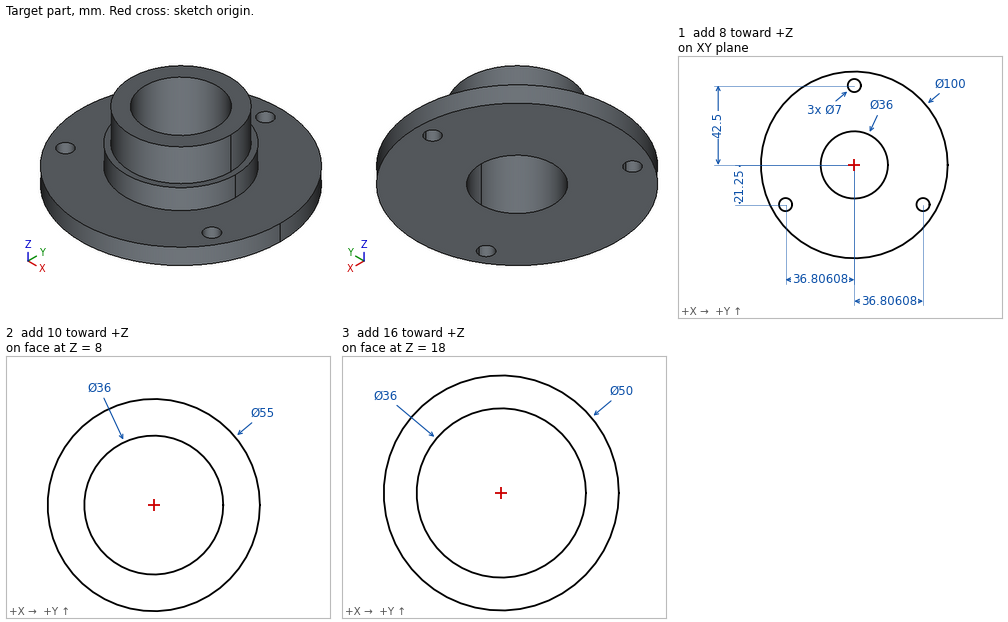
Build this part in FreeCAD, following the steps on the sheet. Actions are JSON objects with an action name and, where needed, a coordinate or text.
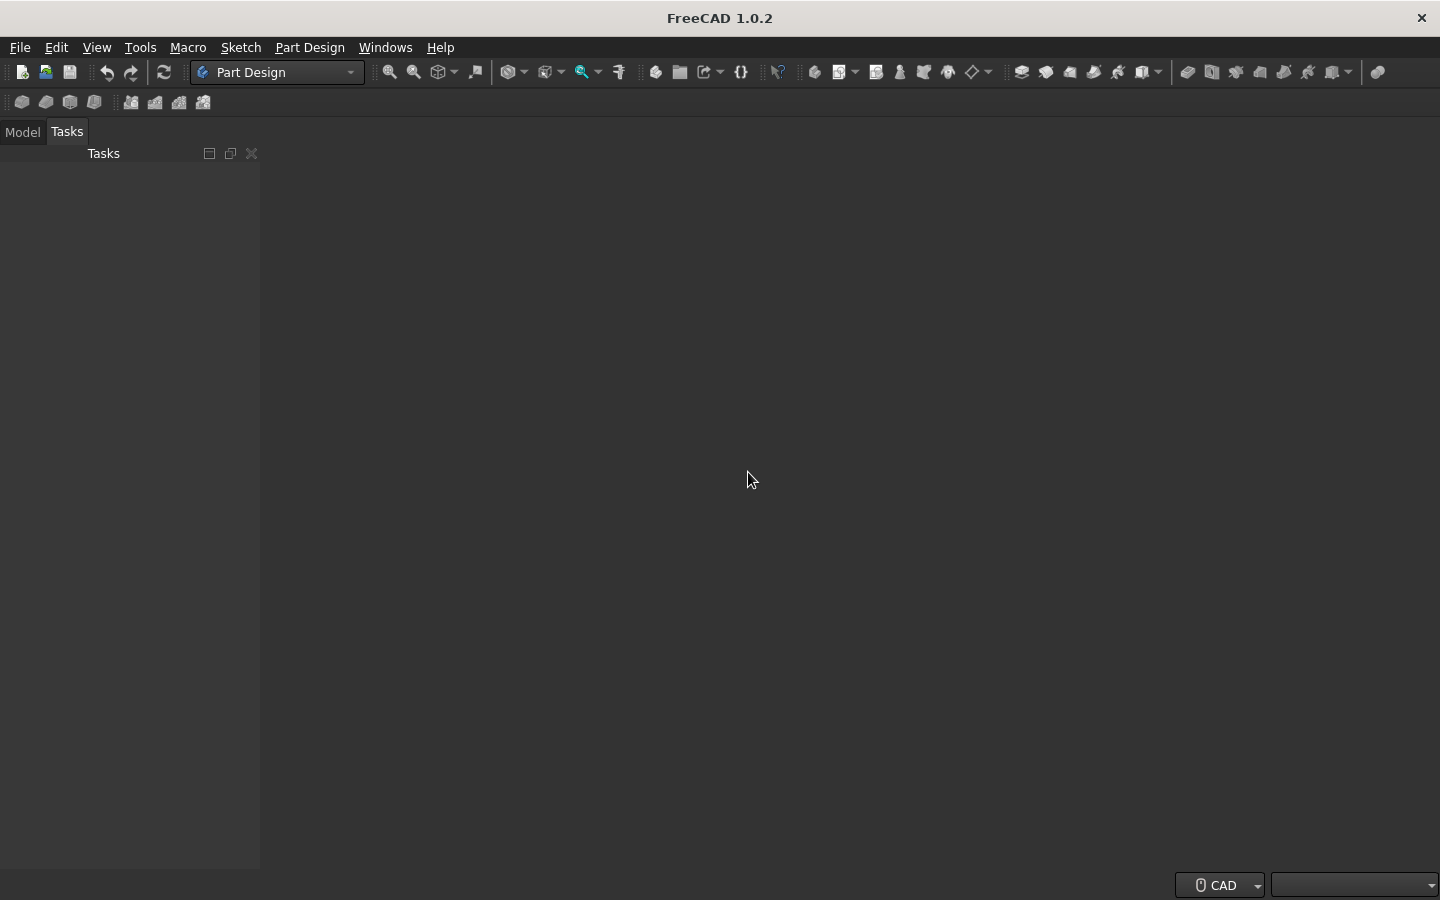
{"action": "left_click", "coordinate": [22, 72]}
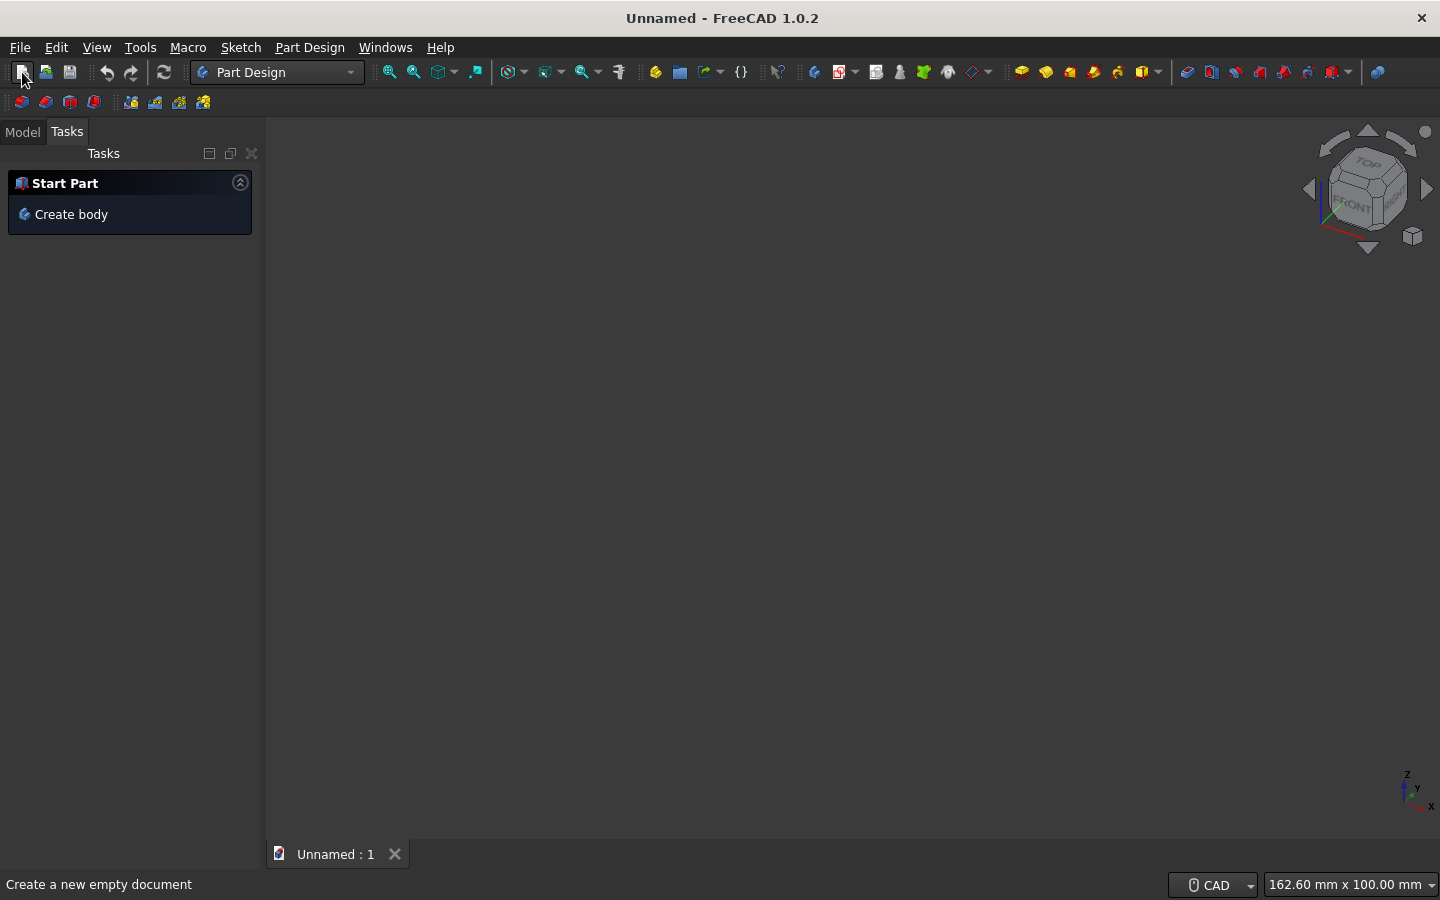
{"action": "left_click", "coordinate": [840, 72]}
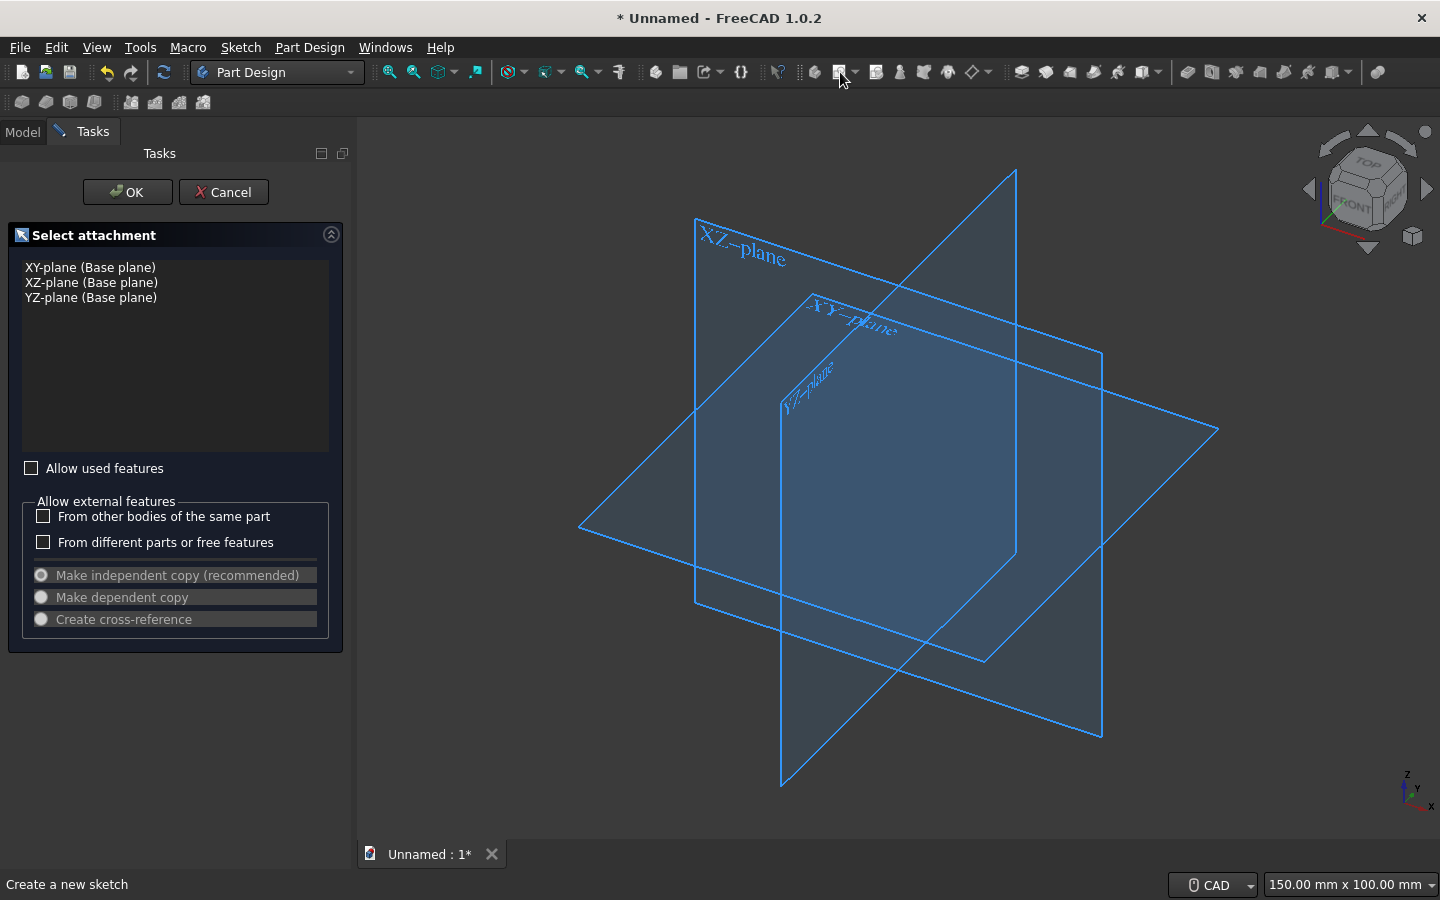
{"action": "left_click", "coordinate": [82, 268]}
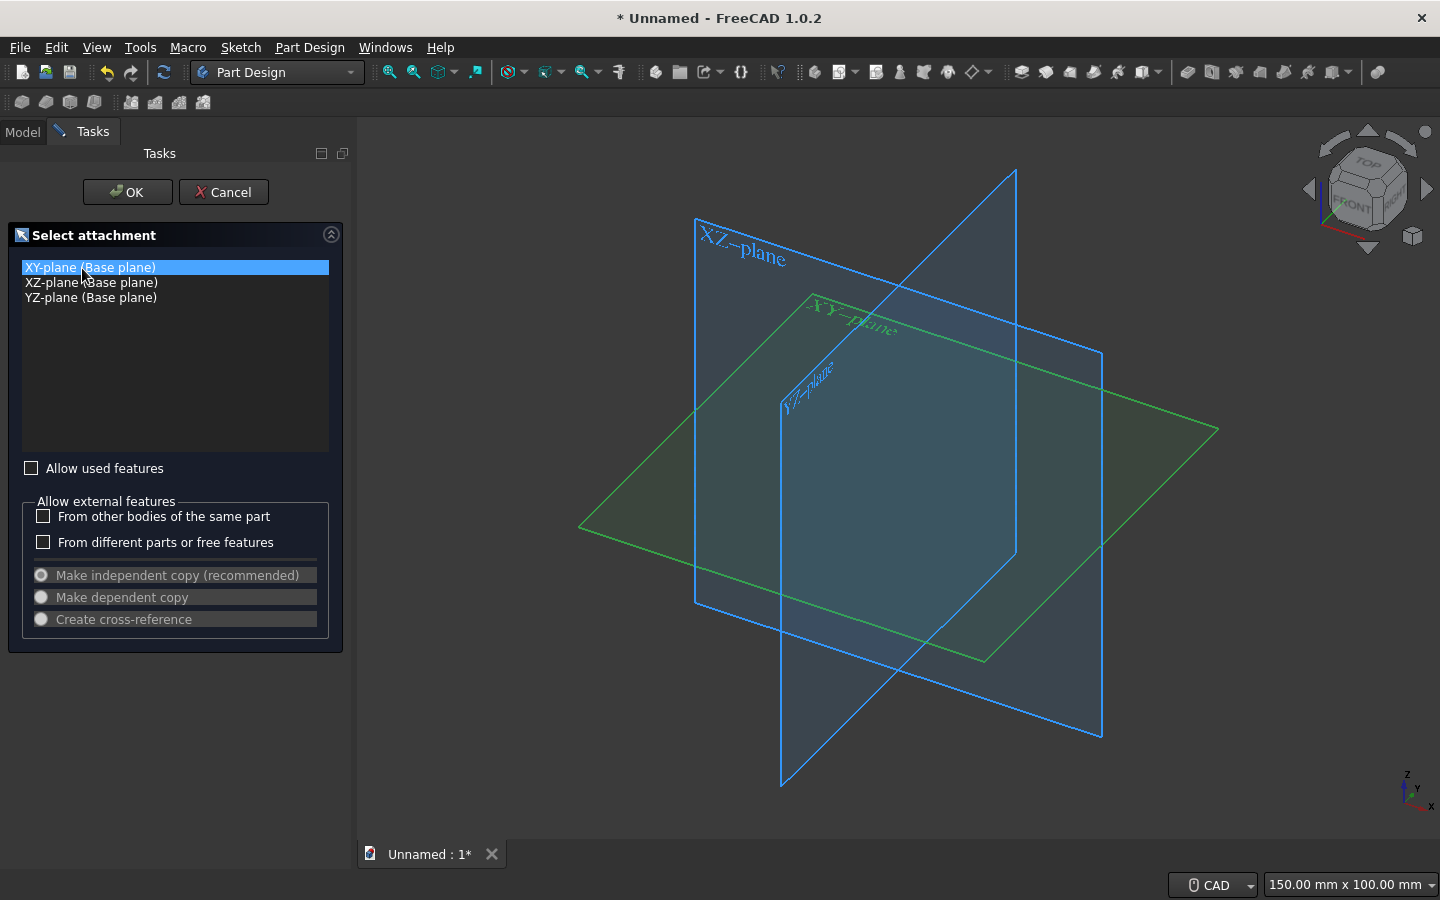
{"action": "left_click", "coordinate": [128, 192]}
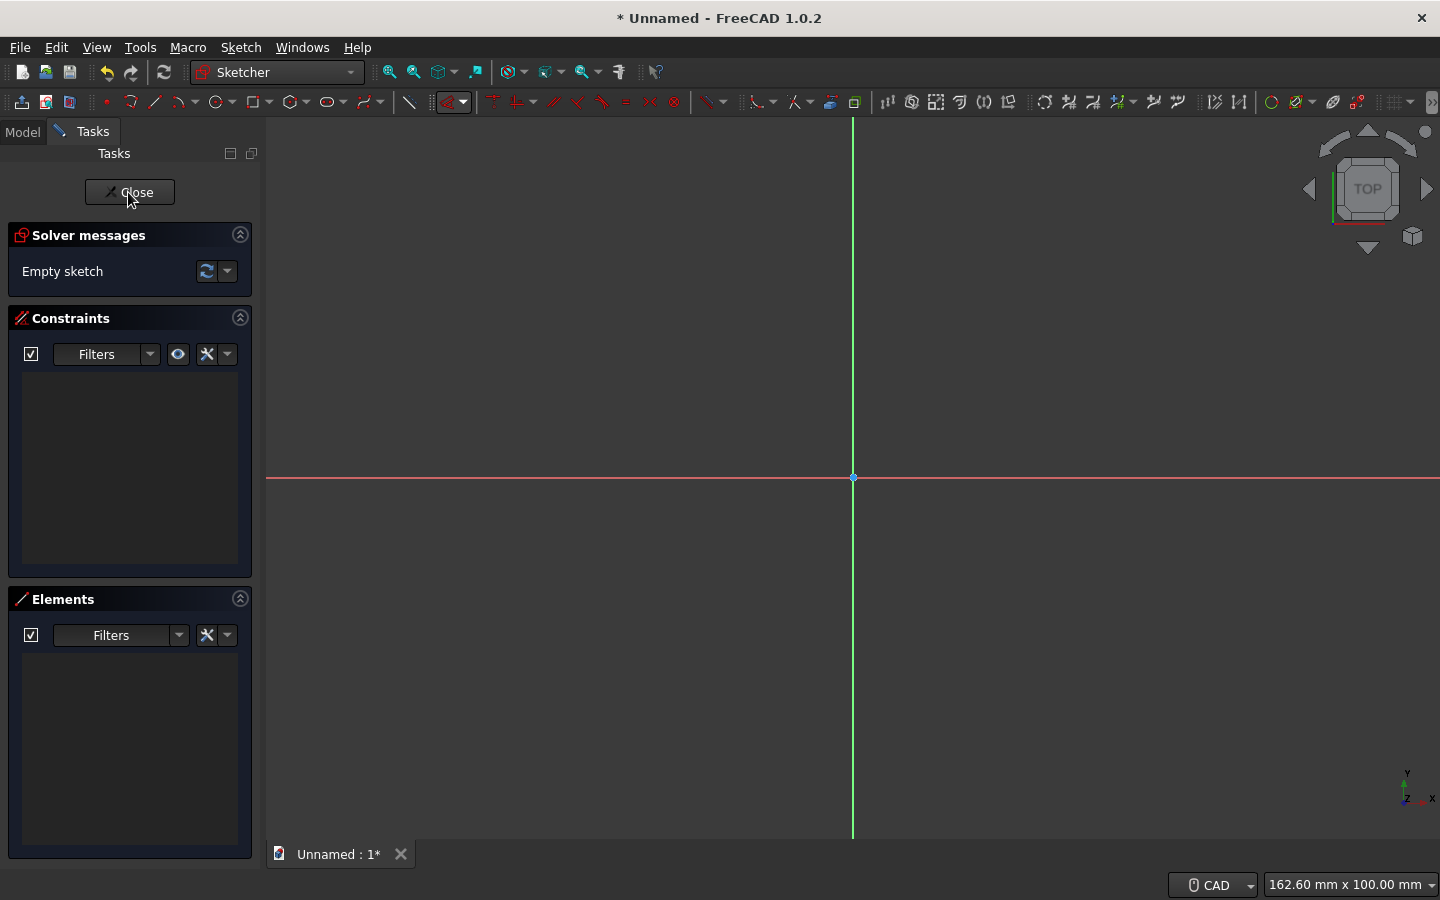
{"action": "scroll", "coordinate": [645, 478], "scroll_direction": "down", "scroll_amount": 2}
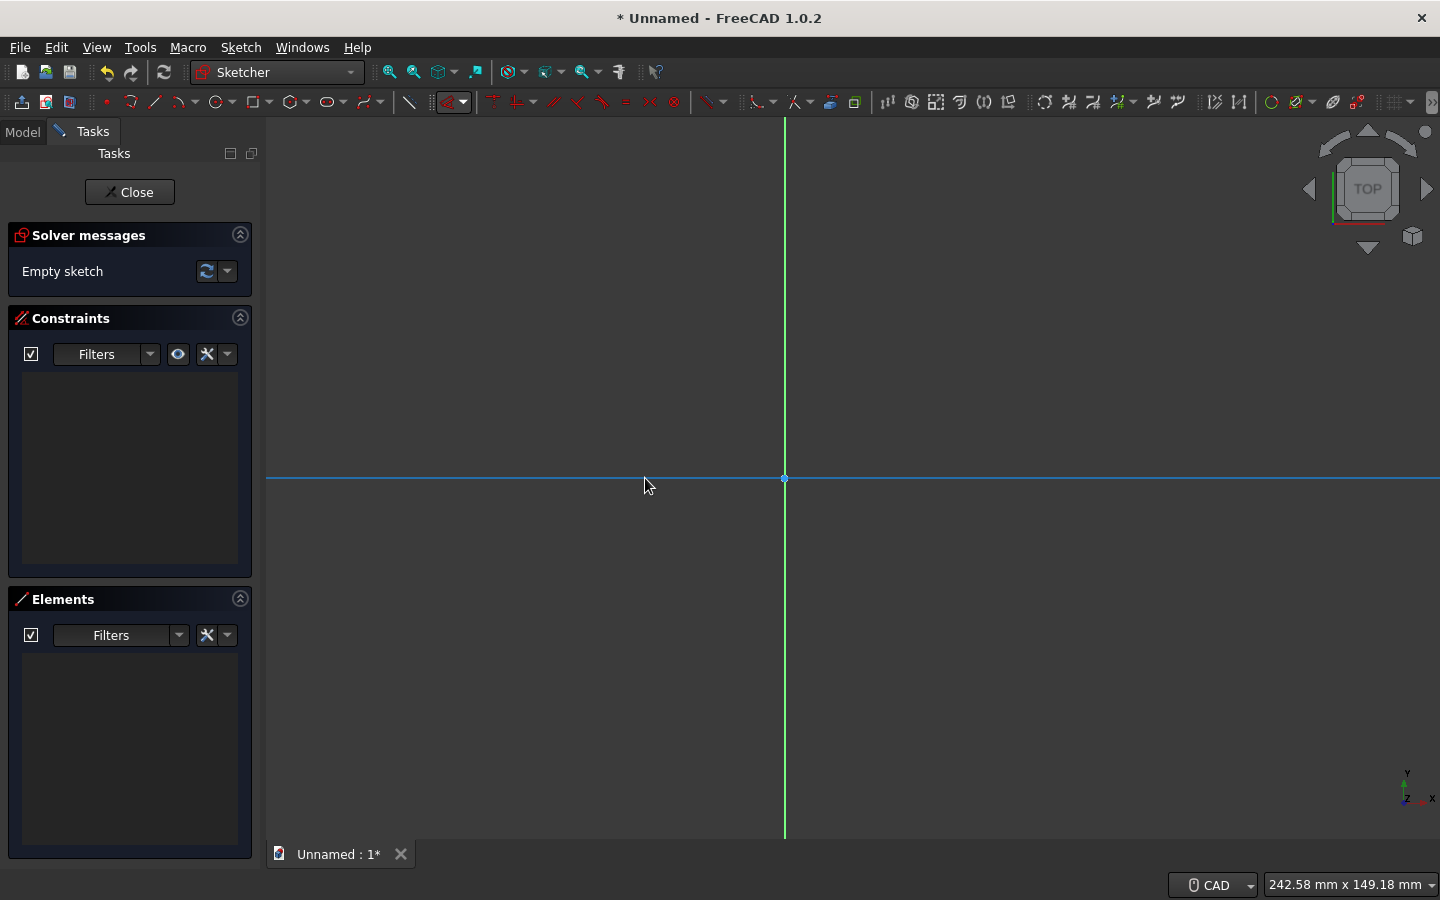
{"action": "left_click", "coordinate": [216, 102]}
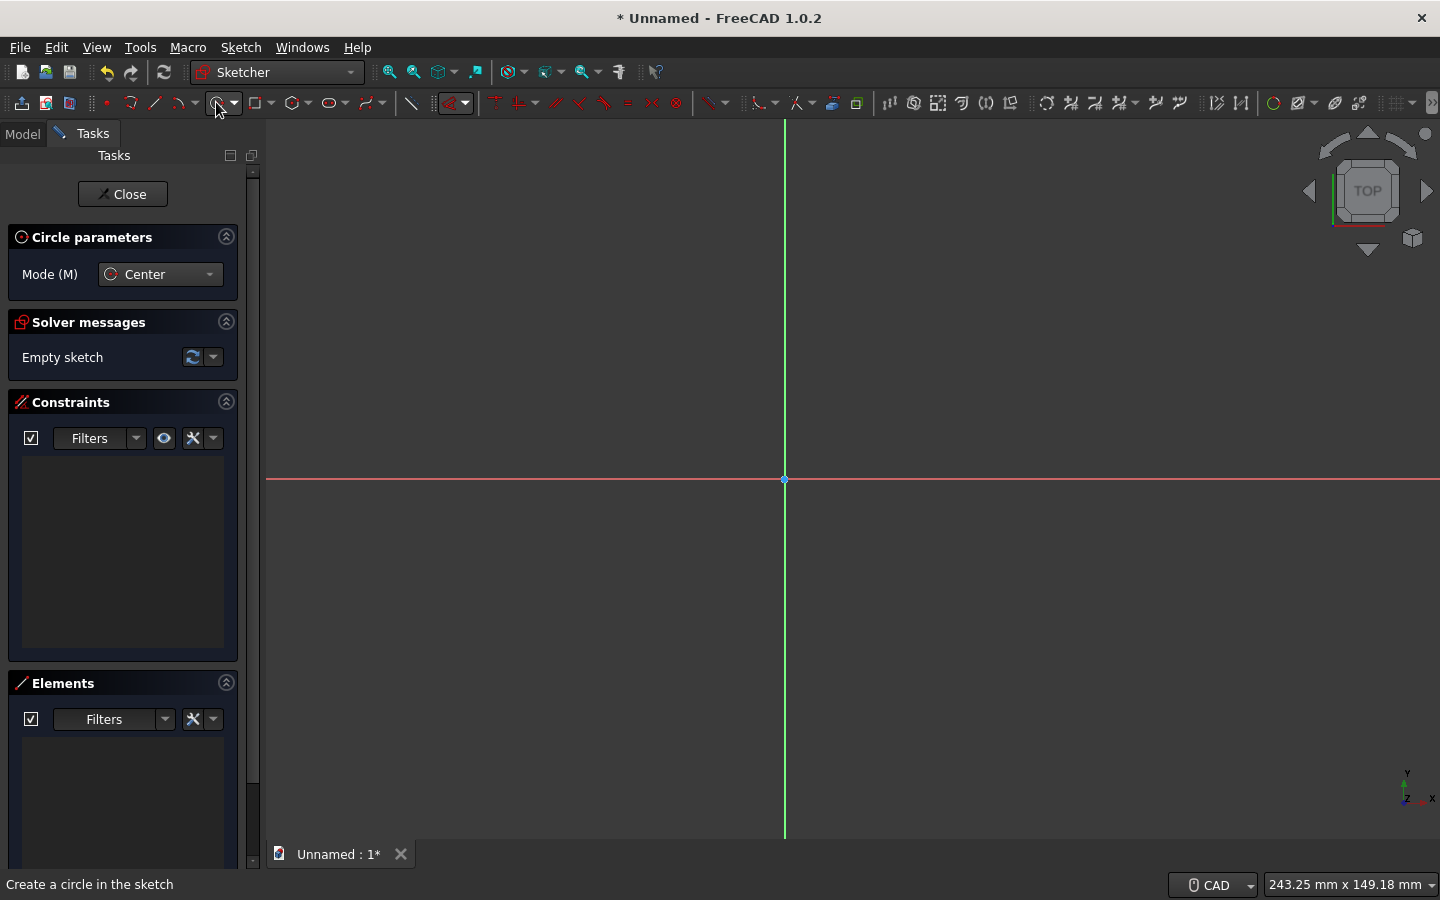
{"action": "left_click", "coordinate": [785, 479]}
{"action": "left_click", "coordinate": [955, 309]}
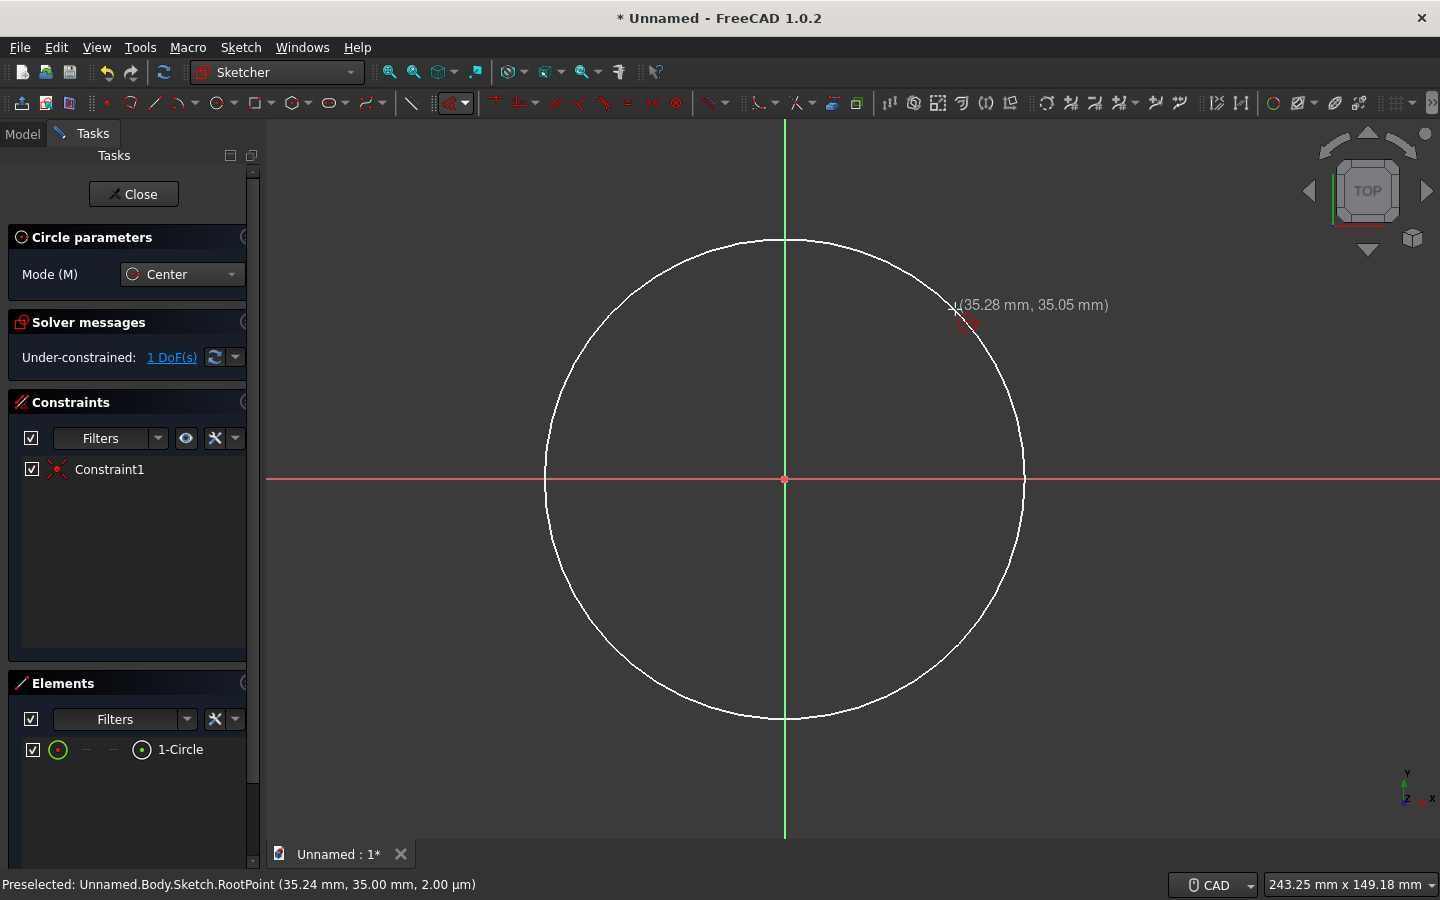
{"action": "scroll", "coordinate": [607, 582], "scroll_direction": "up", "scroll_amount": 2}